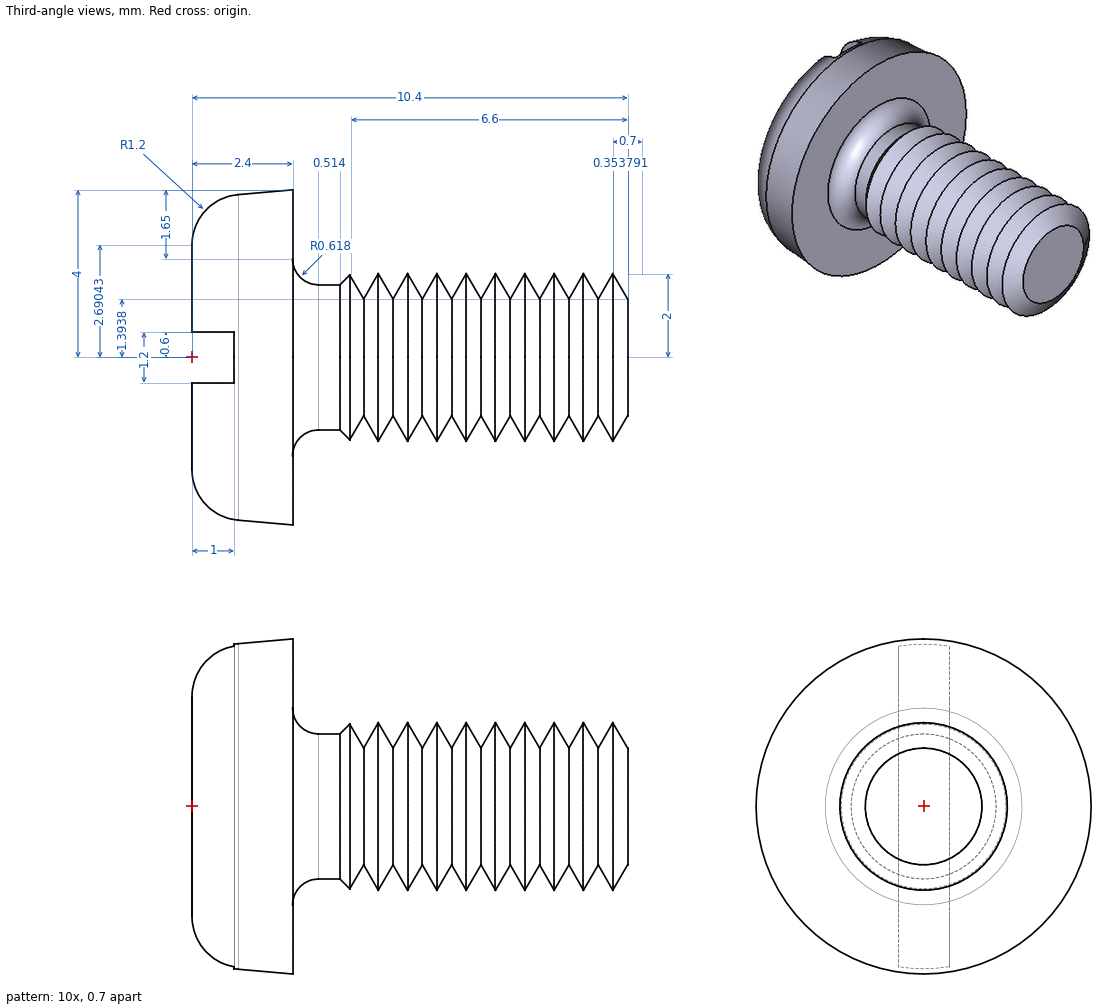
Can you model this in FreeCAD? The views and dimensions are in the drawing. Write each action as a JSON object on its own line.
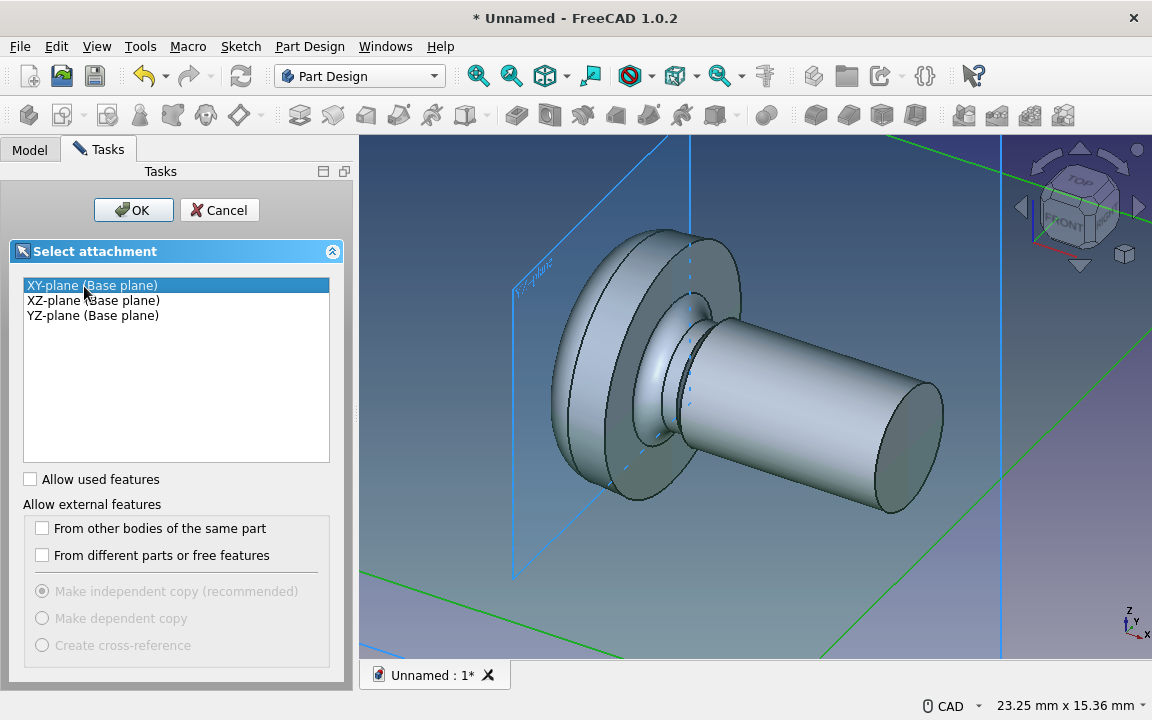
{"action": "left_click", "coordinate": [134, 210]}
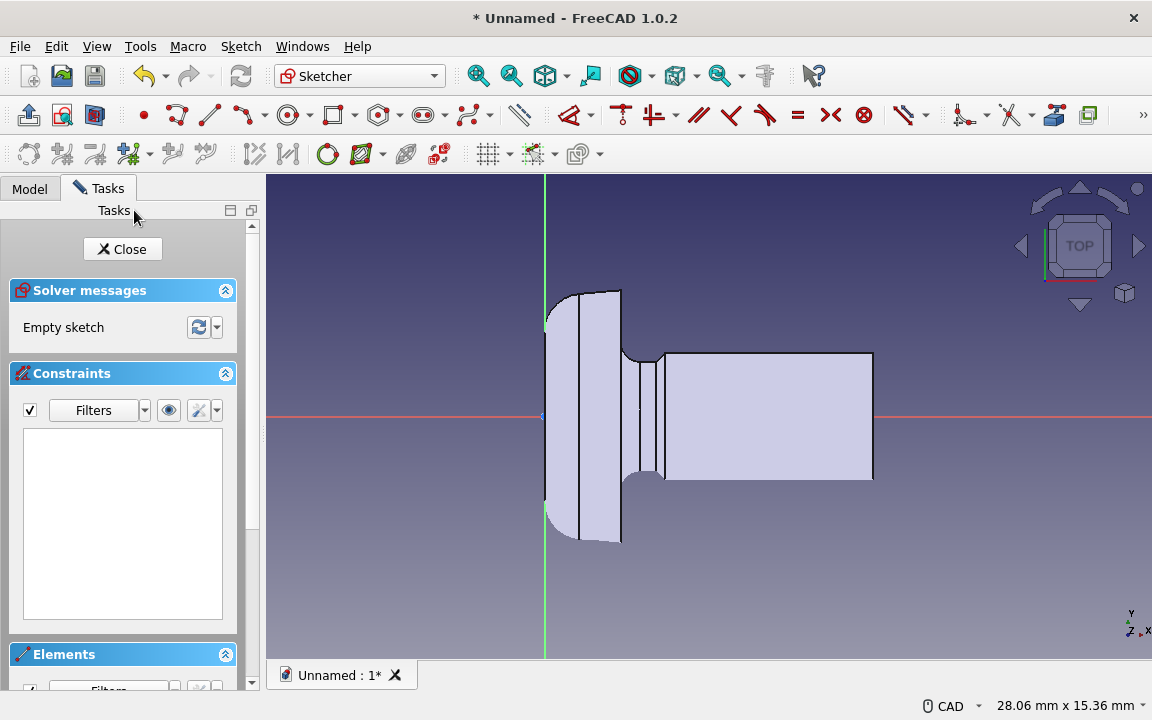
{"action": "left_click", "coordinate": [95, 116]}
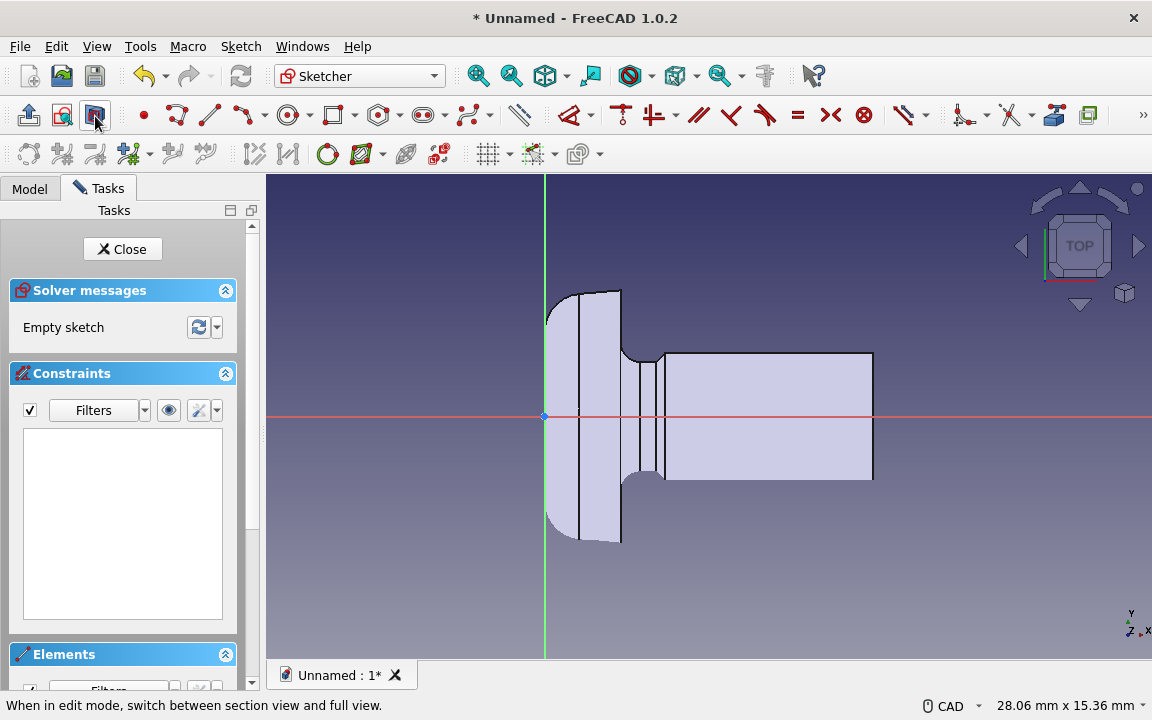
{"action": "scroll", "coordinate": [548, 417], "scroll_direction": "up", "scroll_amount": 10}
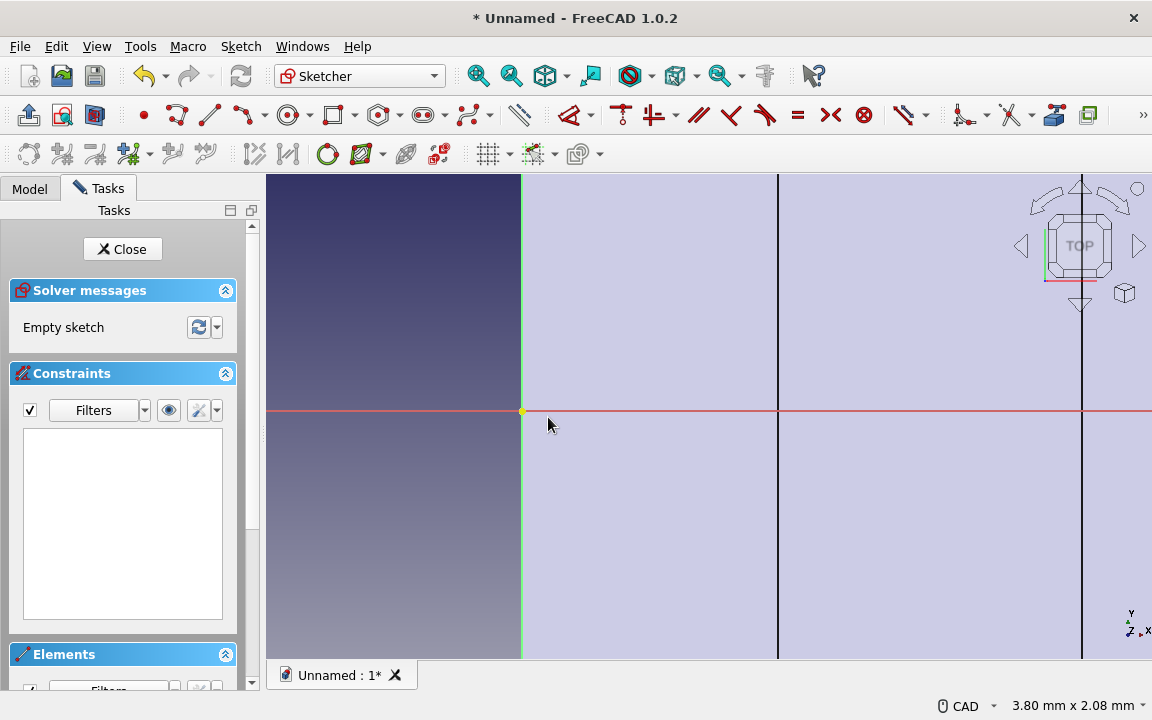
{"action": "left_click", "coordinate": [332, 116]}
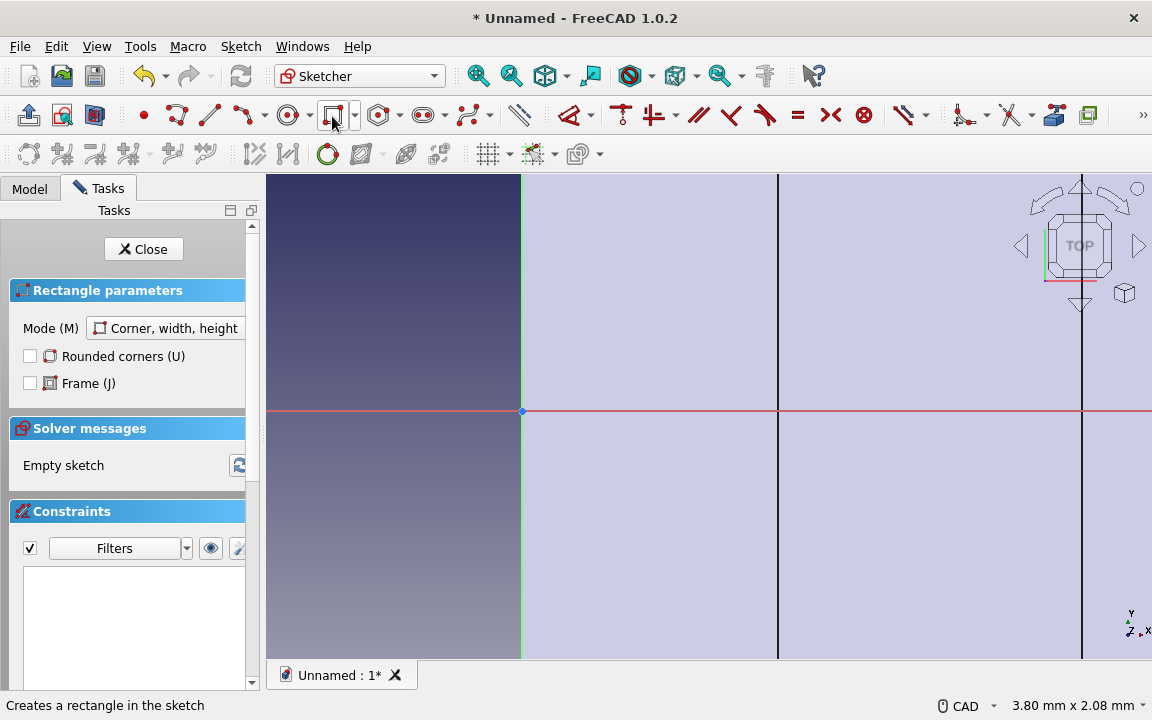
{"action": "left_click", "coordinate": [522, 271]}
{"action": "left_click", "coordinate": [756, 551]}
{"action": "key", "text": "Escape"}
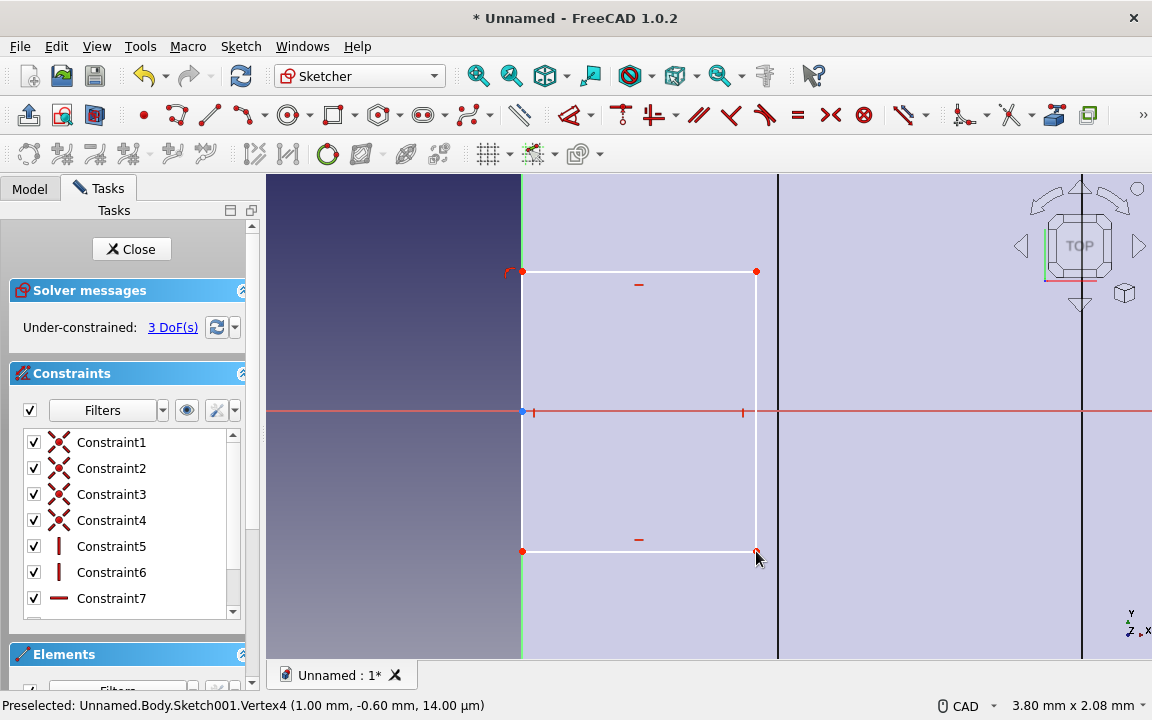
{"action": "left_click", "coordinate": [568, 116]}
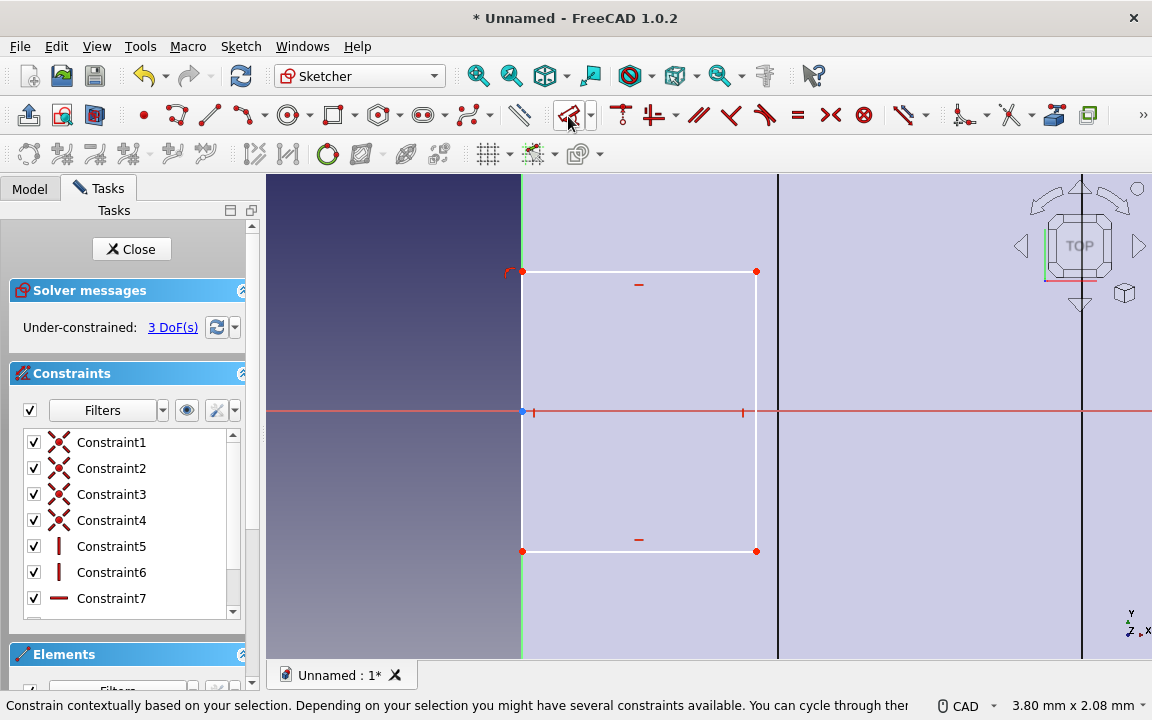
{"action": "left_click", "coordinate": [592, 552]}
{"action": "left_click", "coordinate": [639, 586]}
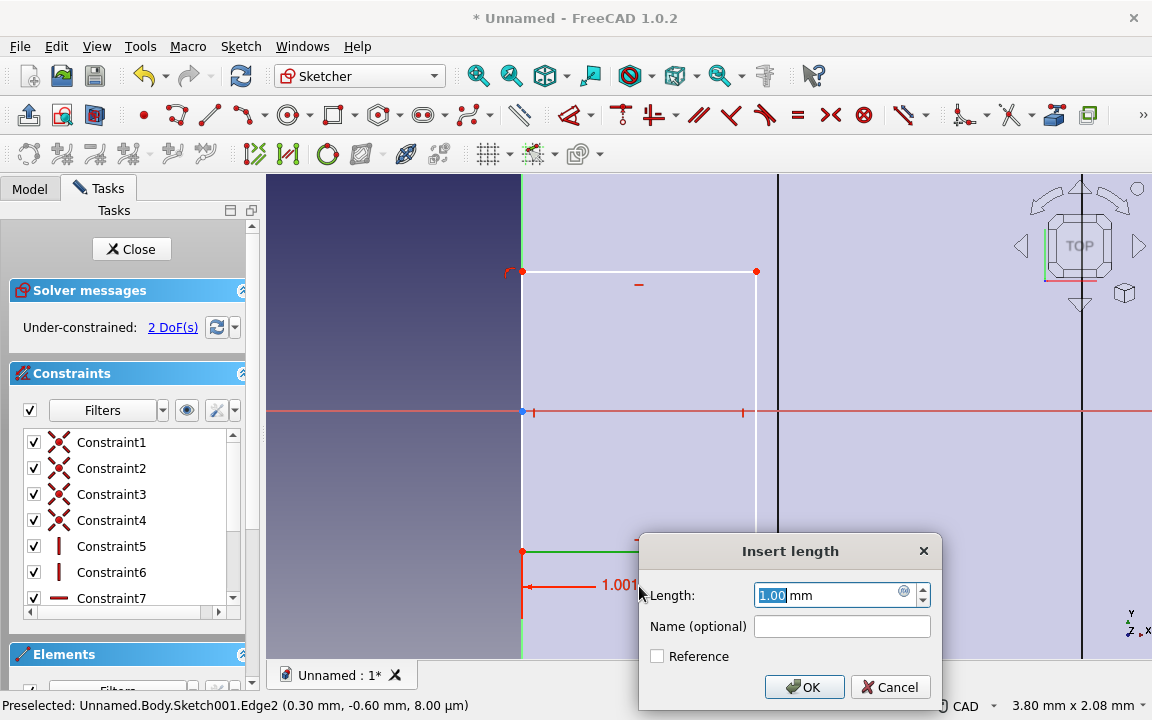
{"action": "type", "text": "1"}
{"action": "key", "text": "Return"}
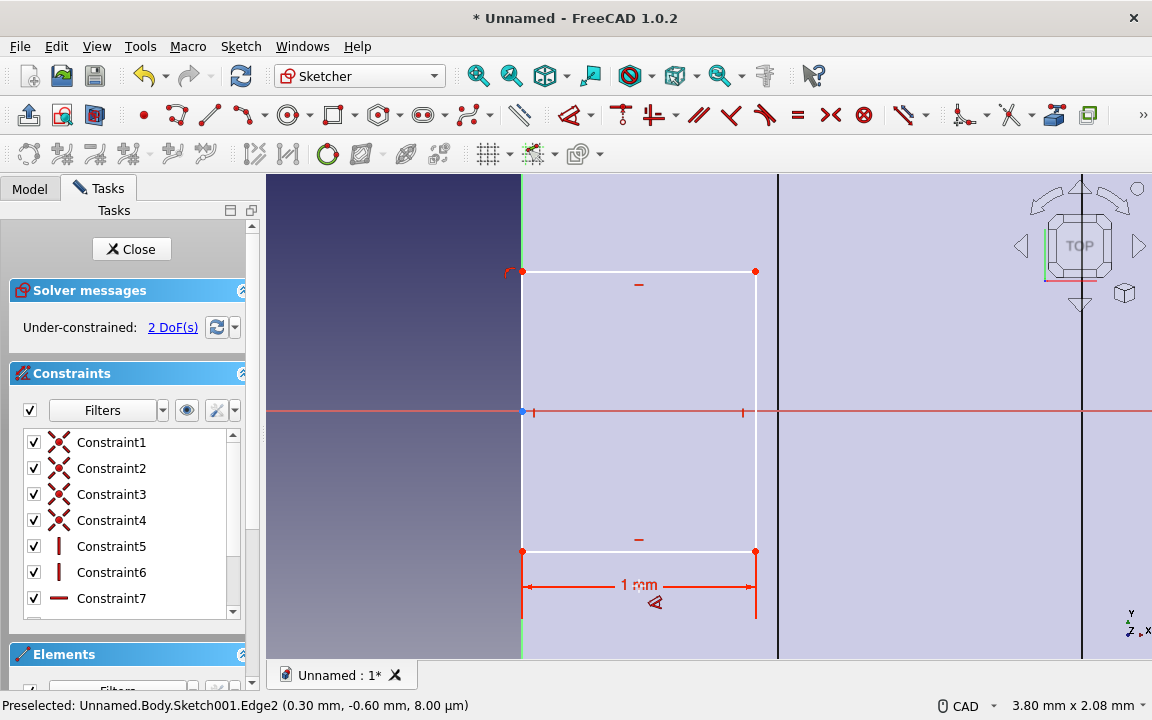
{"action": "left_click", "coordinate": [522, 356]}
{"action": "left_click", "coordinate": [488, 348]}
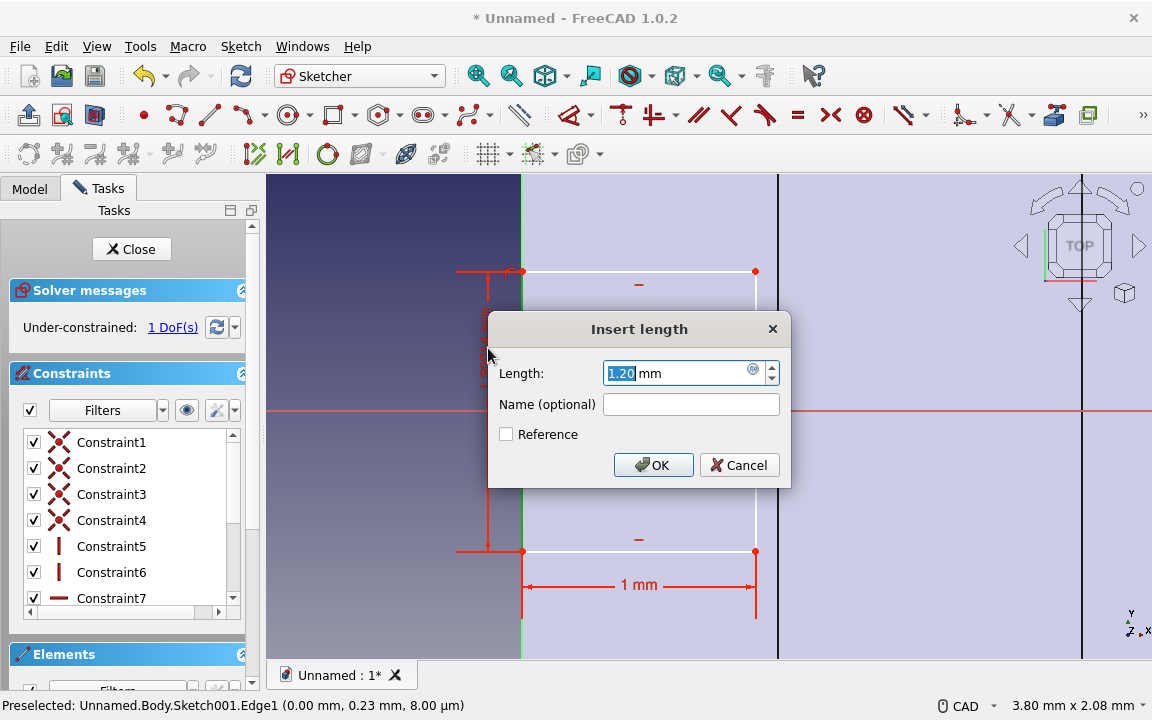
{"action": "type", "text": "1.2"}
{"action": "key", "text": "Return"}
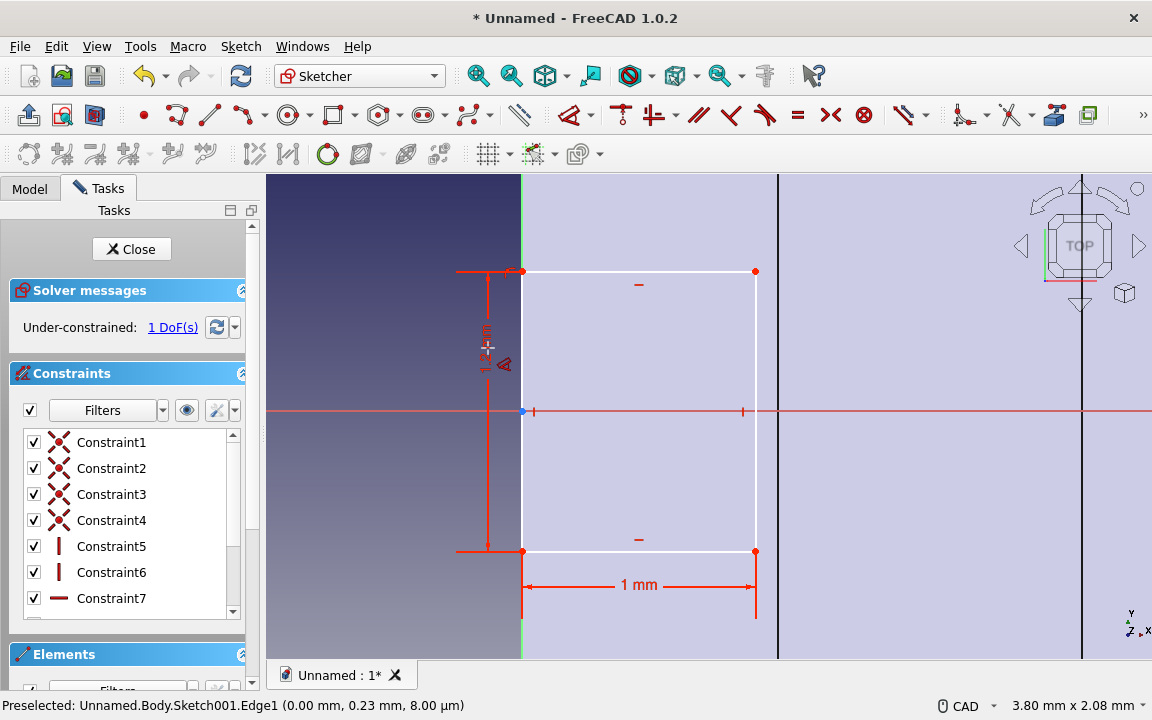
{"action": "left_click", "coordinate": [522, 272]}
{"action": "left_click", "coordinate": [488, 310]}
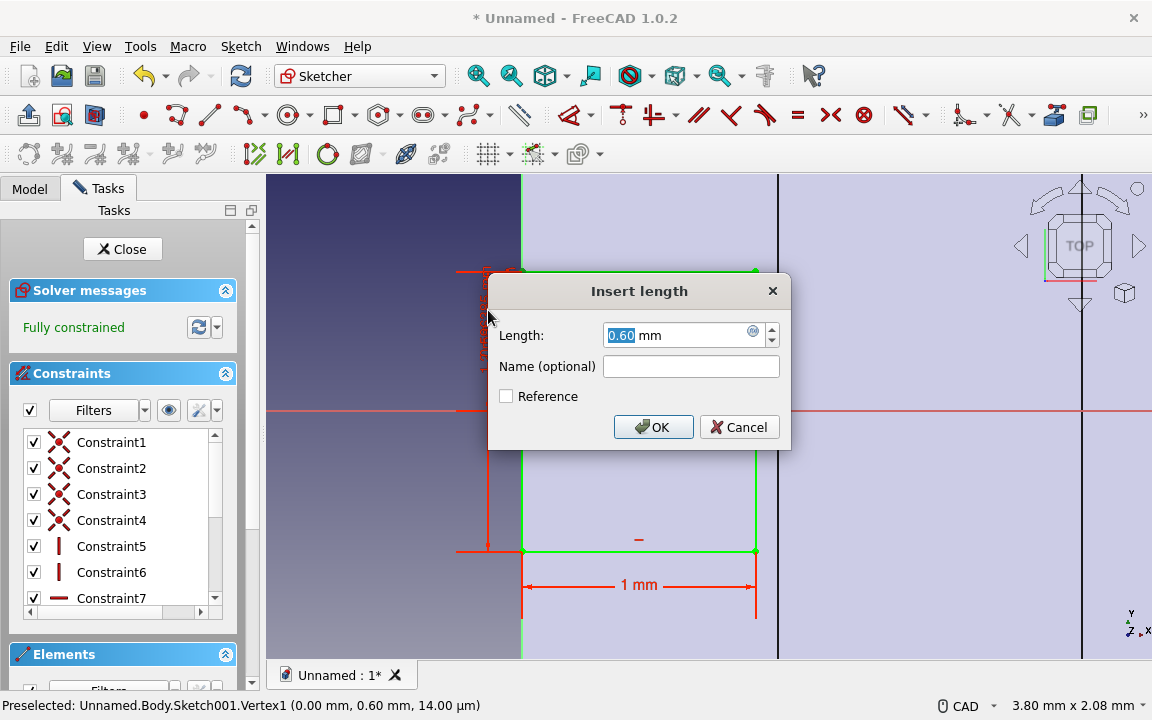
{"action": "type", "text": "0.6"}
{"action": "key", "text": "Return"}
{"action": "key", "text": "Escape"}